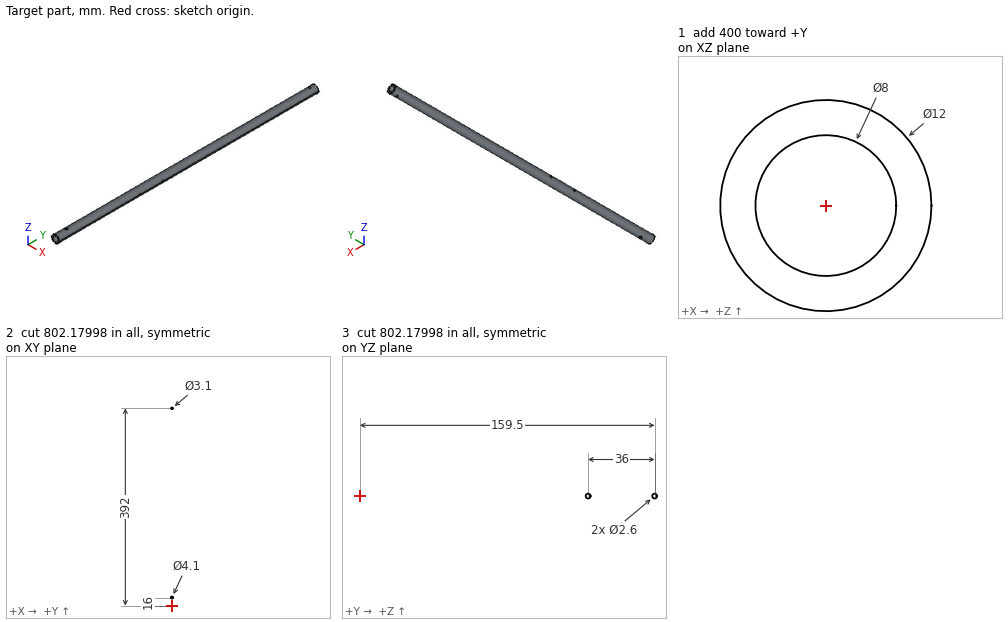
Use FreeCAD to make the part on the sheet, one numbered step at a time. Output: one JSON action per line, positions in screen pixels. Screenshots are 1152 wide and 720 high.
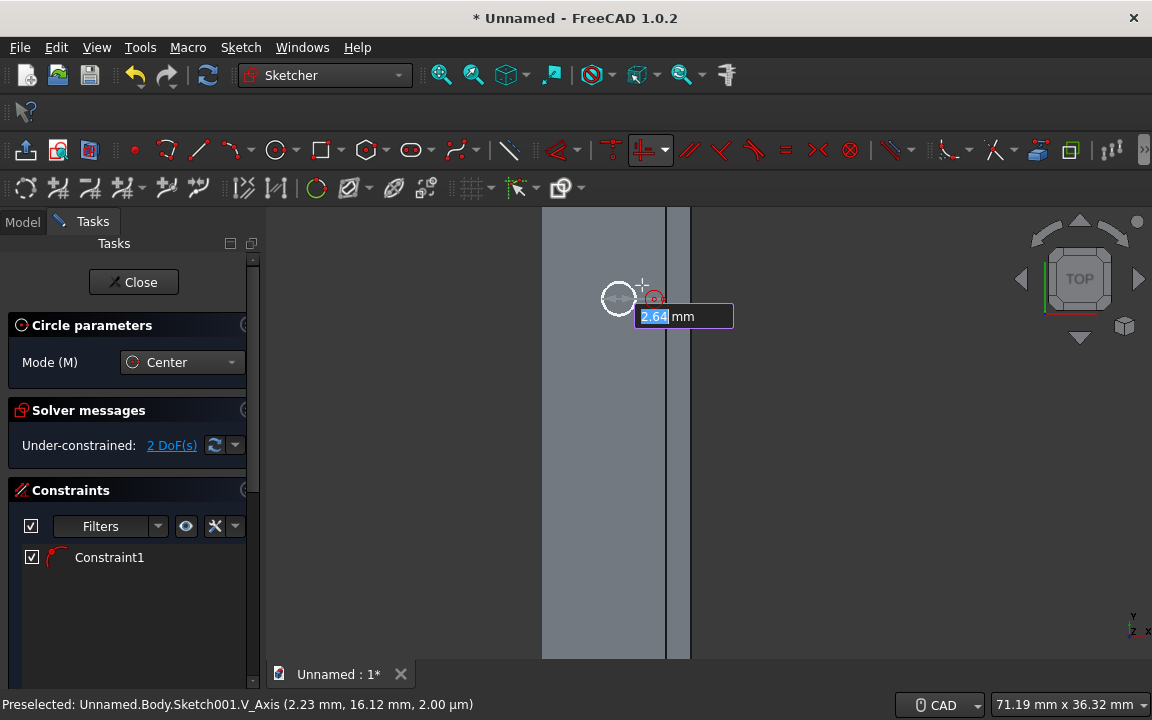
{"action": "left_click", "coordinate": [635, 279]}
{"action": "key", "text": "Escape"}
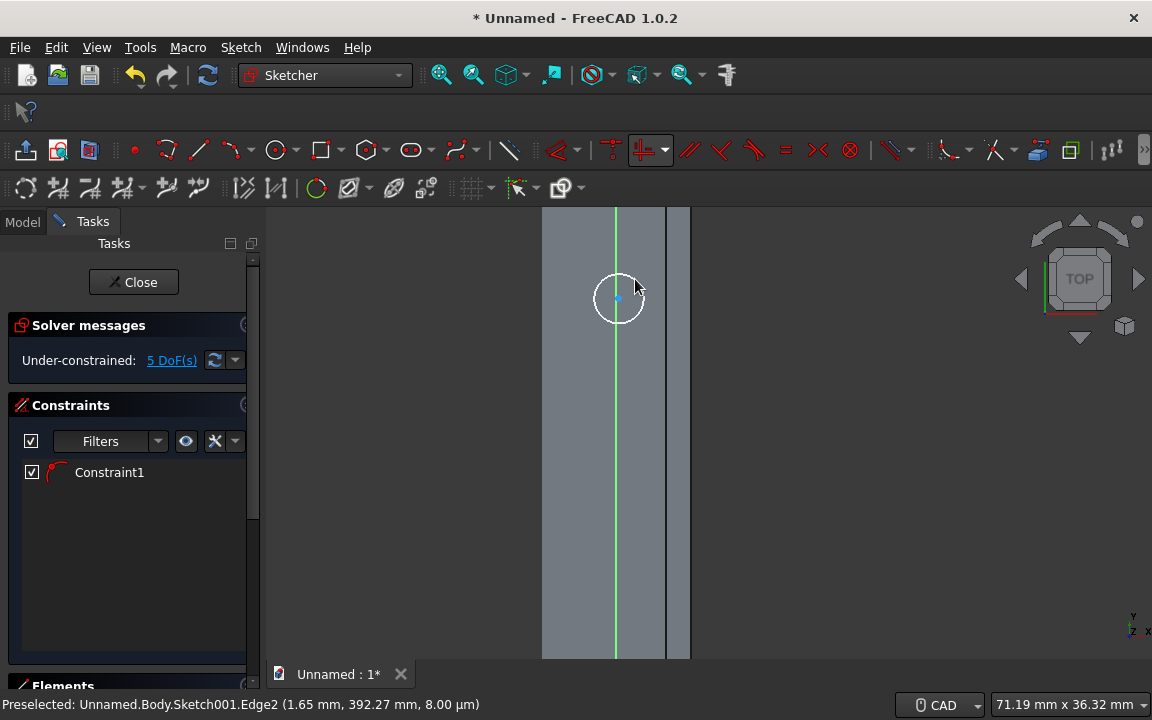
{"action": "scroll", "coordinate": [642, 285], "scroll_direction": "down", "scroll_amount": 14}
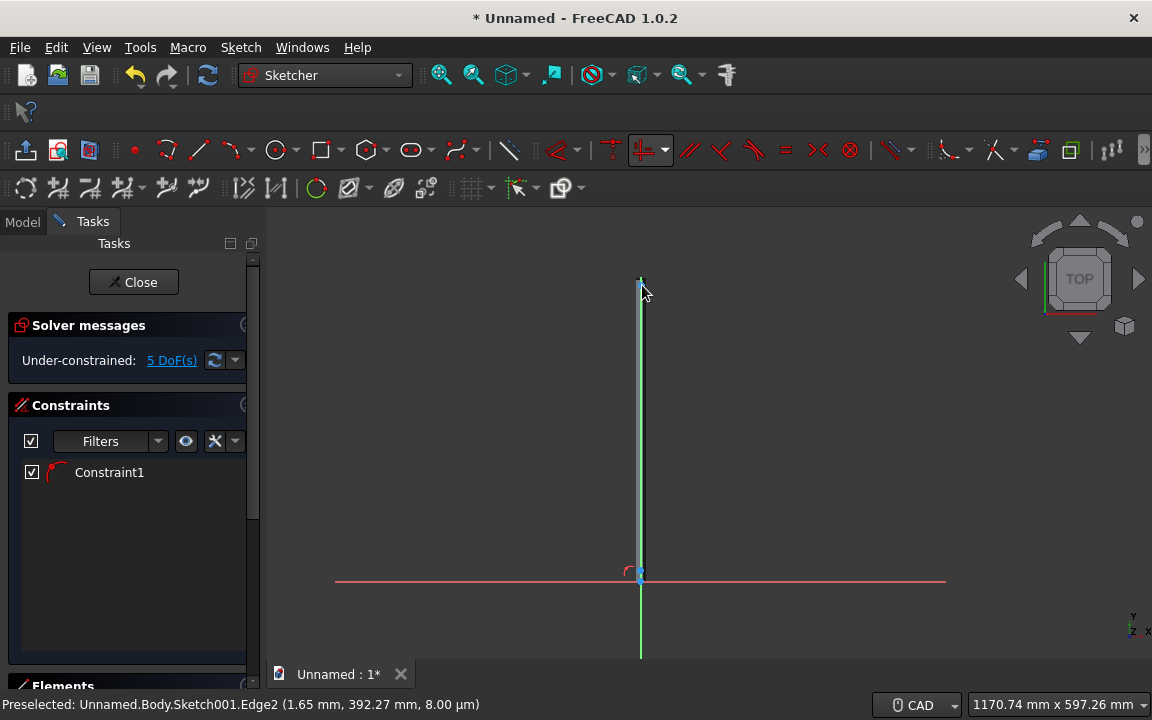
{"action": "left_click", "coordinate": [641, 286]}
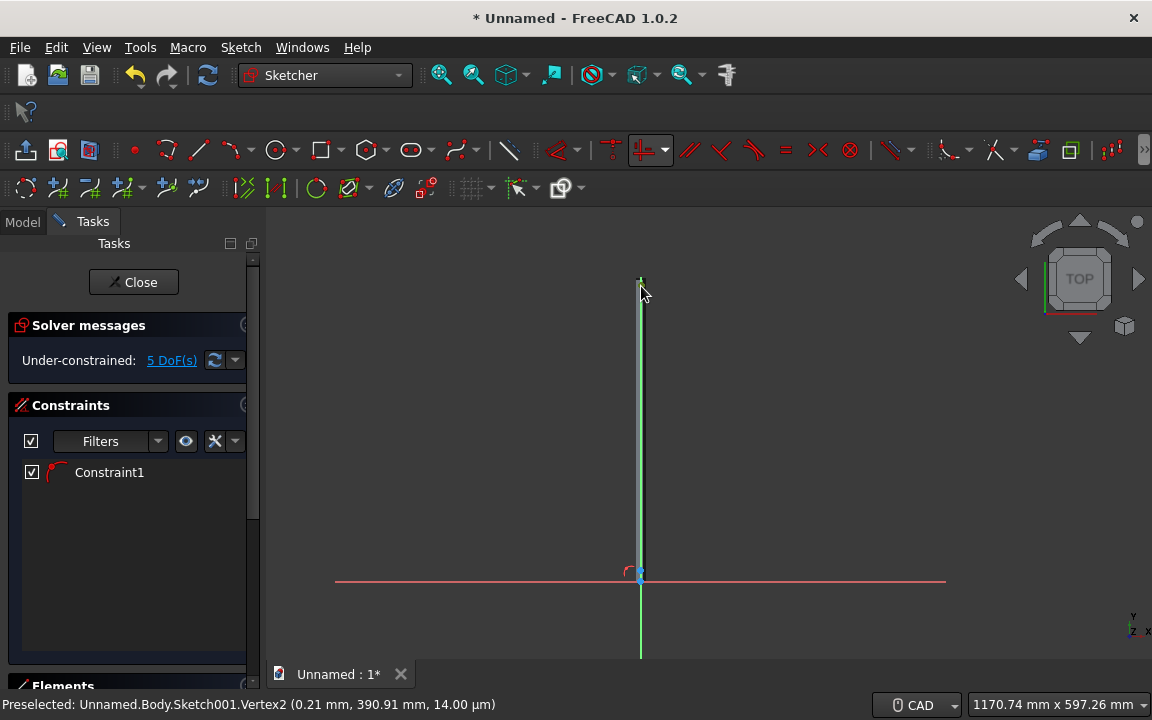
{"action": "left_click", "coordinate": [641, 518]}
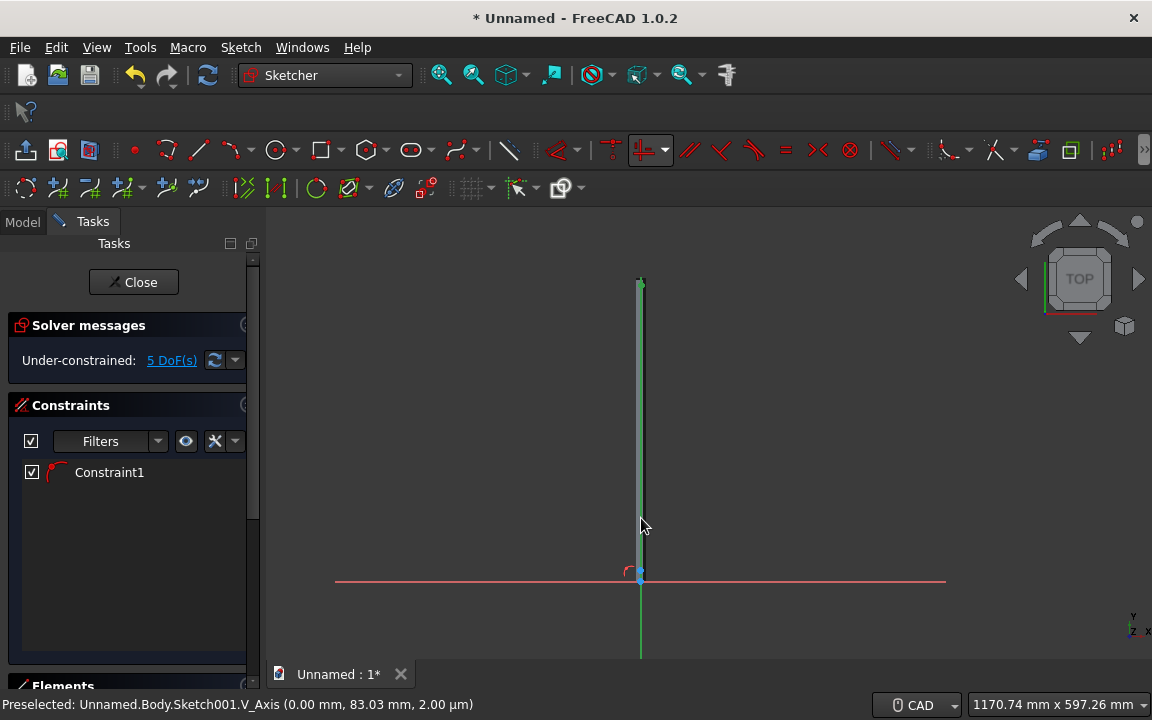
{"action": "left_click", "coordinate": [612, 150]}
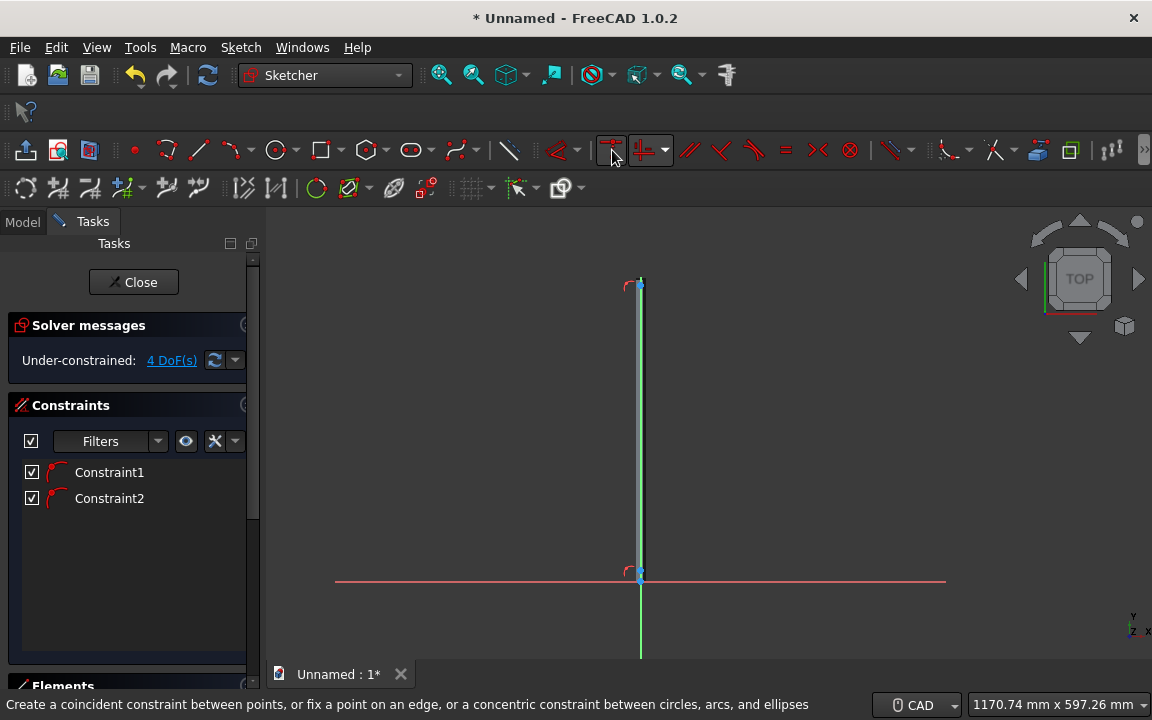
{"action": "left_click", "coordinate": [556, 150]}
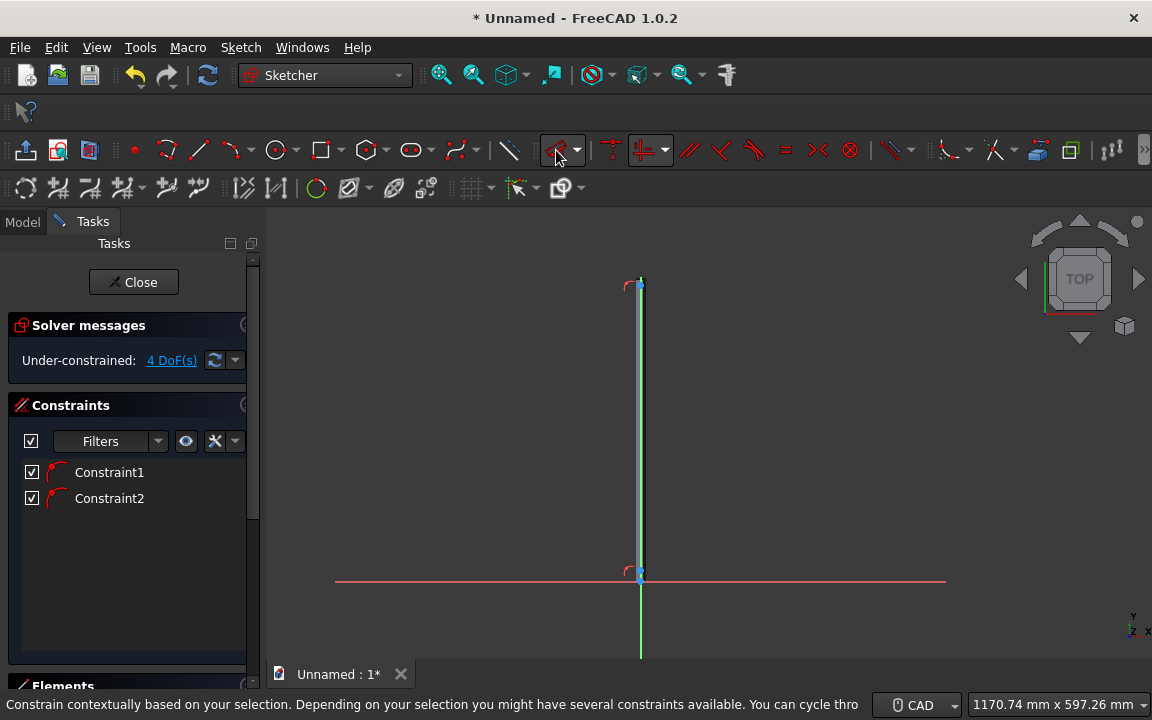
{"action": "scroll", "coordinate": [641, 569], "scroll_direction": "up", "scroll_amount": 13}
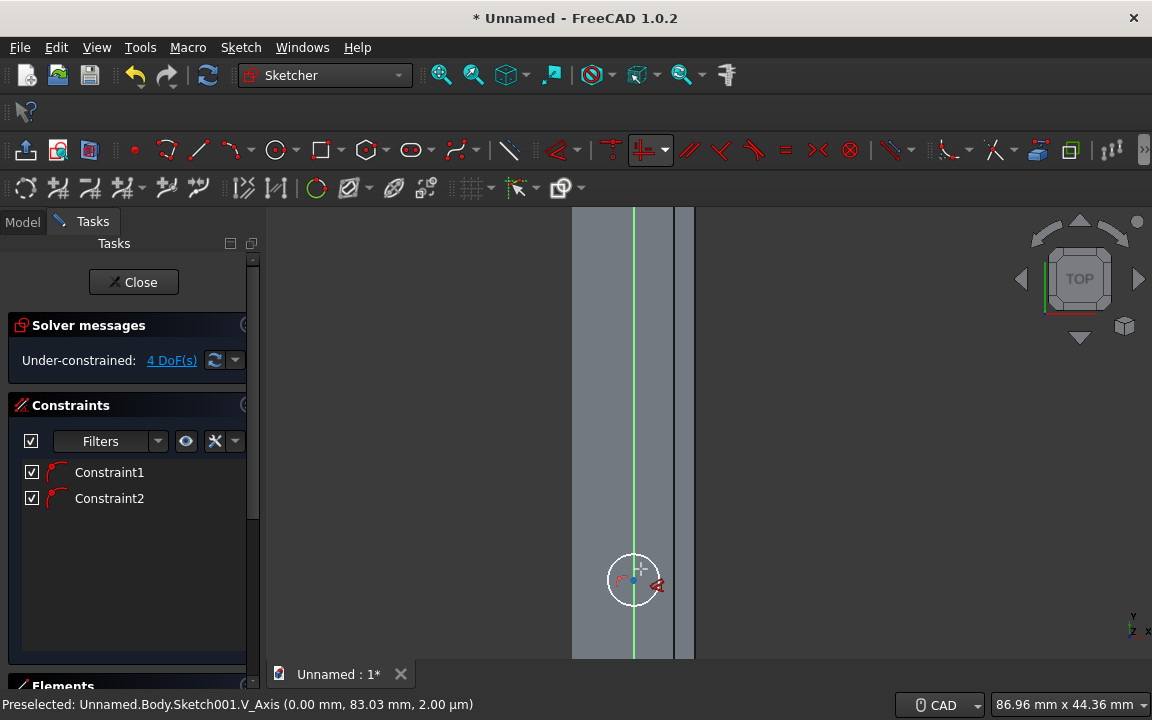
{"action": "left_click", "coordinate": [634, 554]}
{"action": "left_click", "coordinate": [662, 530]}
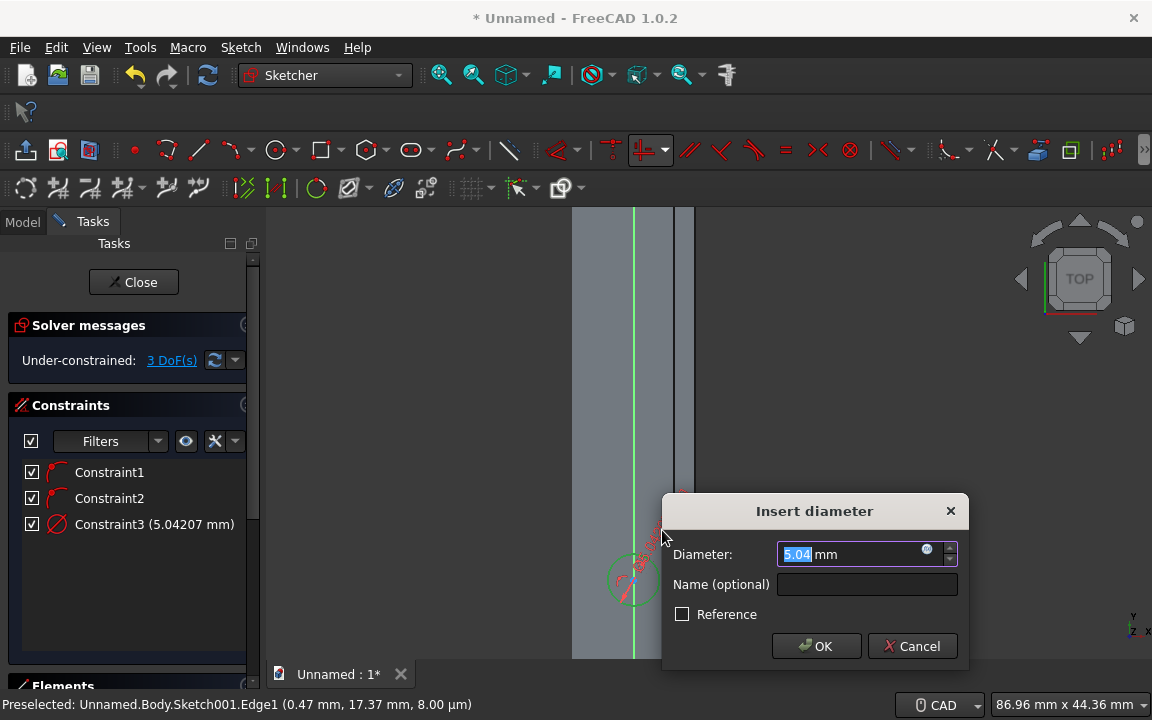
{"action": "type", "text": "4.1"}
{"action": "key", "text": "Return"}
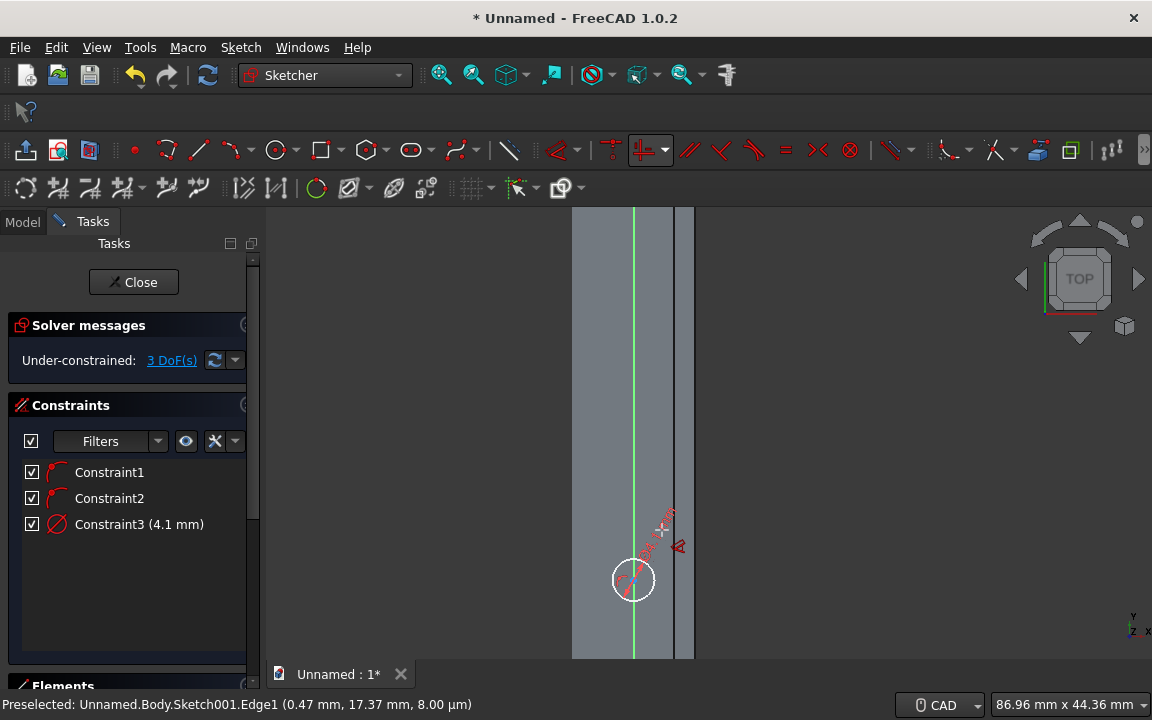
{"action": "scroll", "coordinate": [641, 570], "scroll_direction": "down", "scroll_amount": 13}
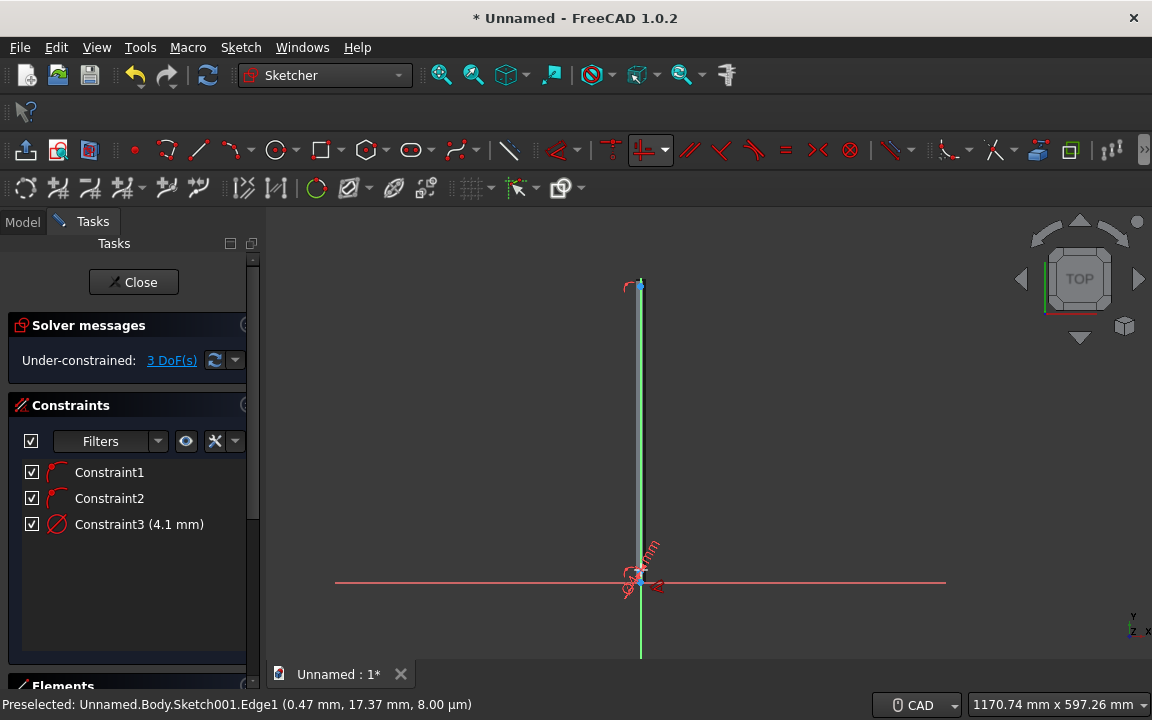
{"action": "scroll", "coordinate": [642, 286], "scroll_direction": "up", "scroll_amount": 15}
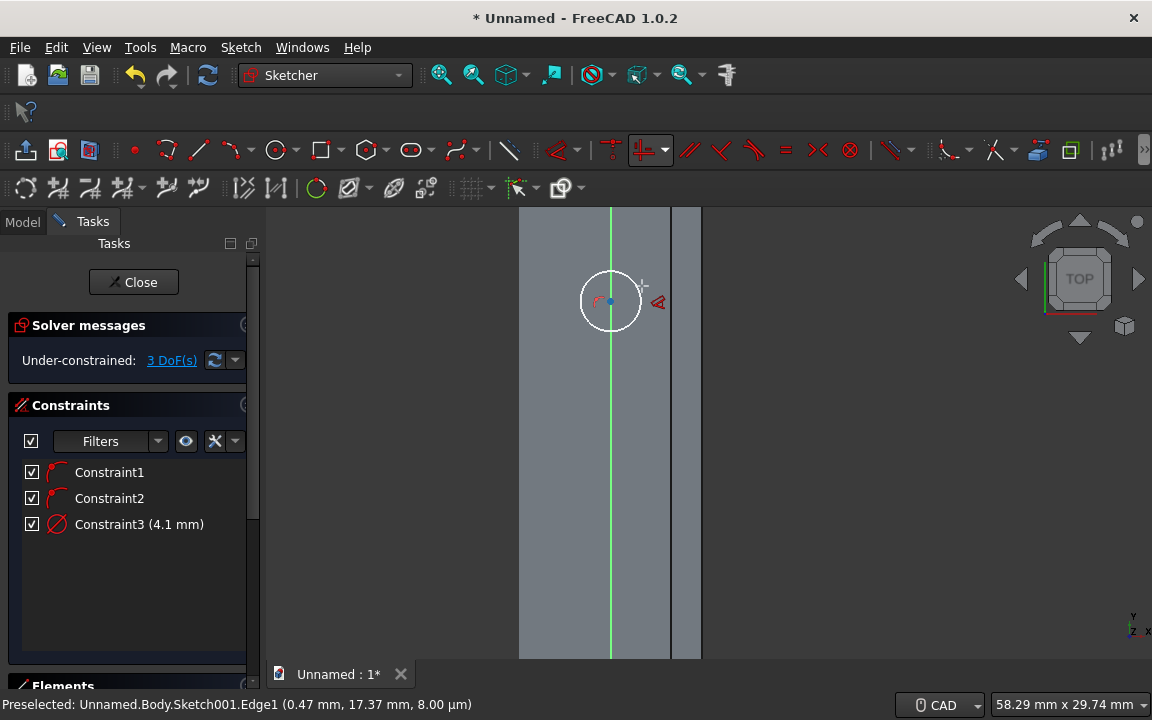
{"action": "left_click", "coordinate": [632, 280]}
{"action": "left_click", "coordinate": [655, 257]}